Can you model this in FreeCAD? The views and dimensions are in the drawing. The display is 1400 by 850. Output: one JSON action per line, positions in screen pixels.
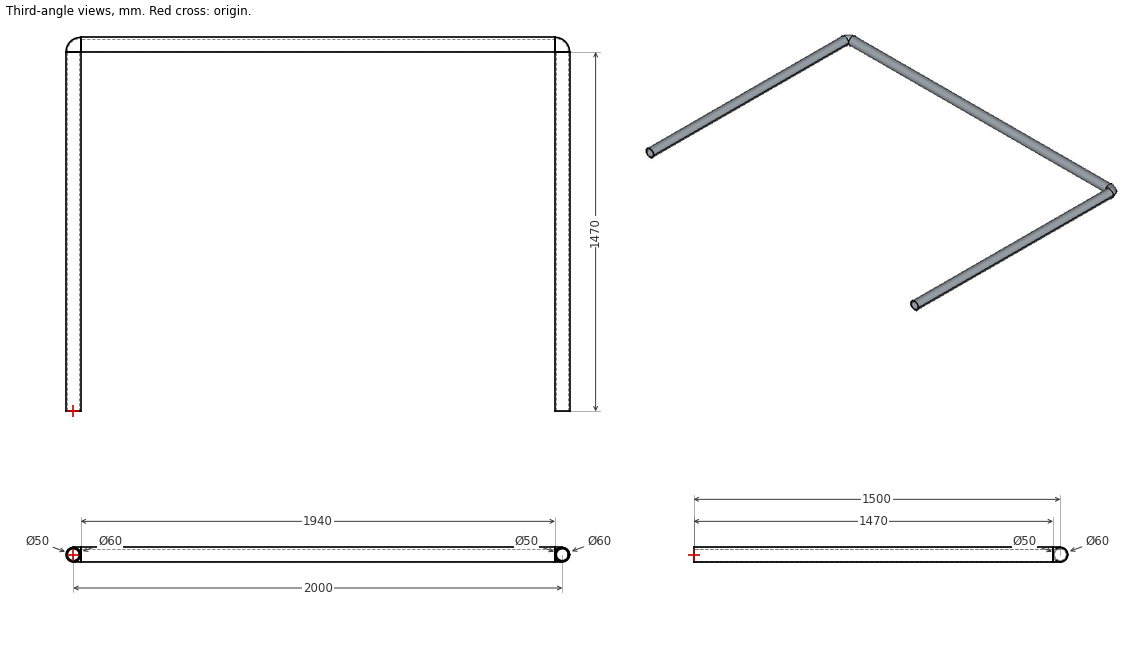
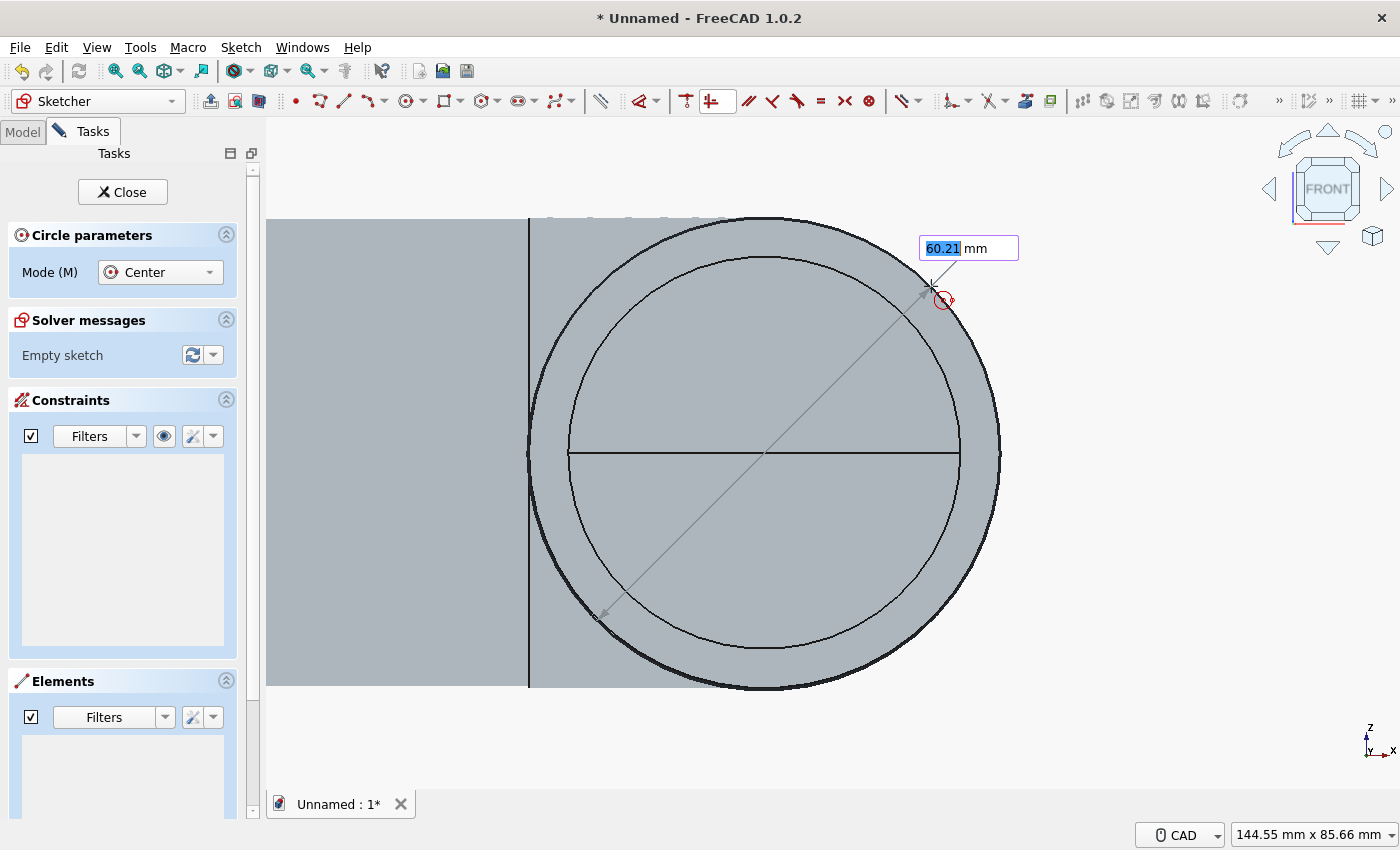
{"action": "type", "text": "60"}
{"action": "key", "text": "Return"}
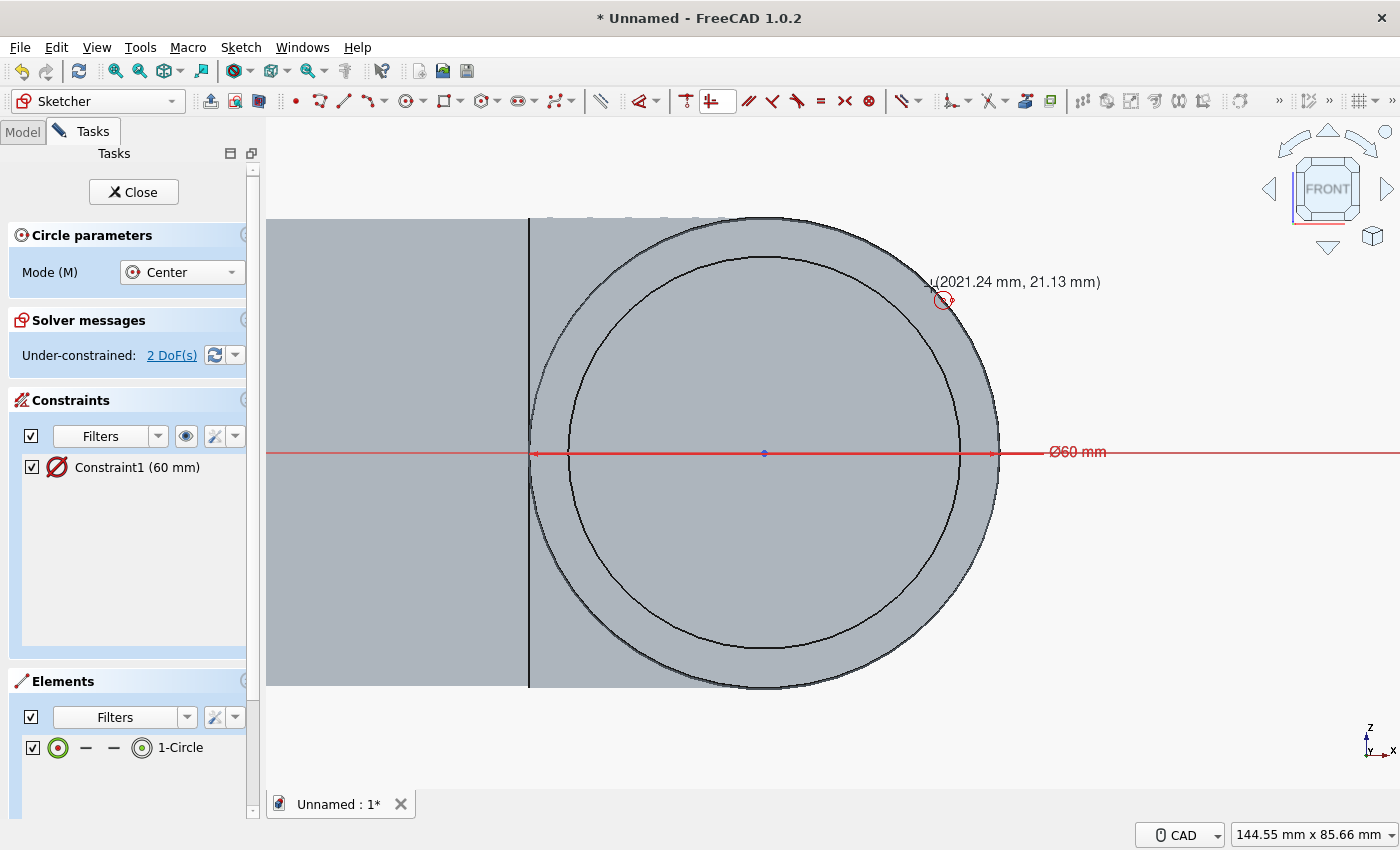
{"action": "left_click", "coordinate": [764, 454]}
{"action": "mouse_move", "coordinate": [903, 314]}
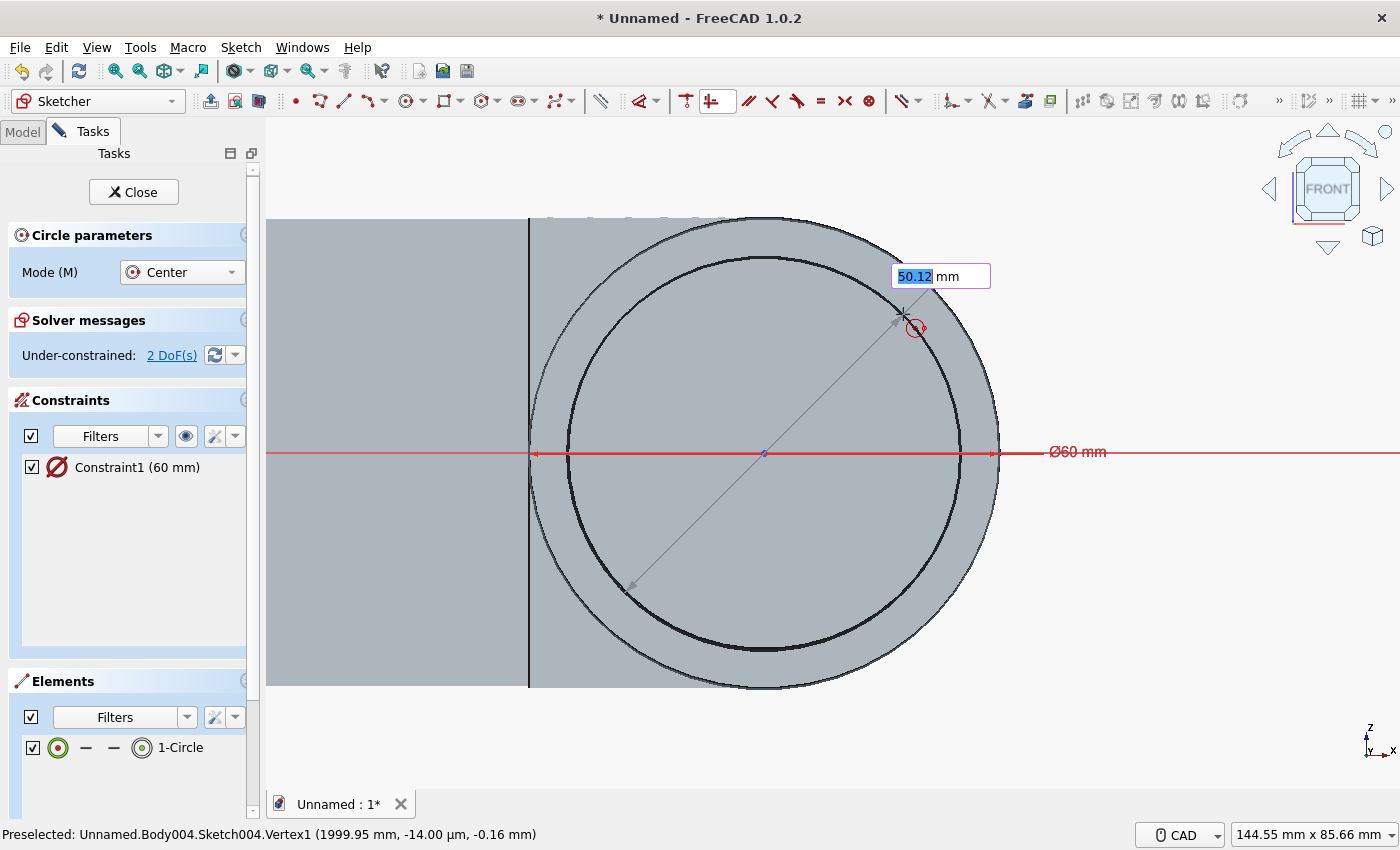
{"action": "type", "text": "50"}
{"action": "key", "text": "Return"}
{"action": "key", "text": "Escape"}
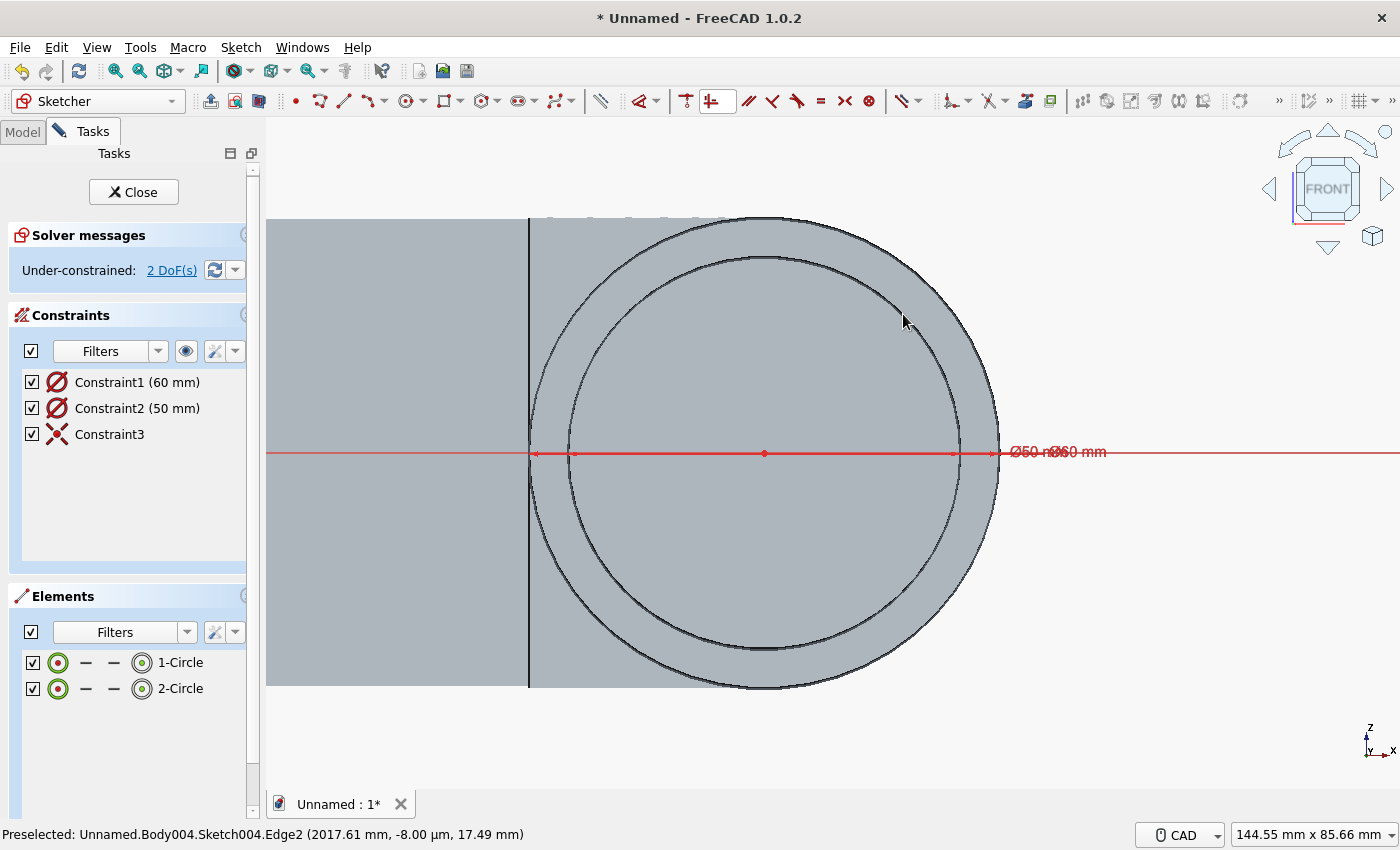
{"action": "left_click", "coordinate": [764, 454]}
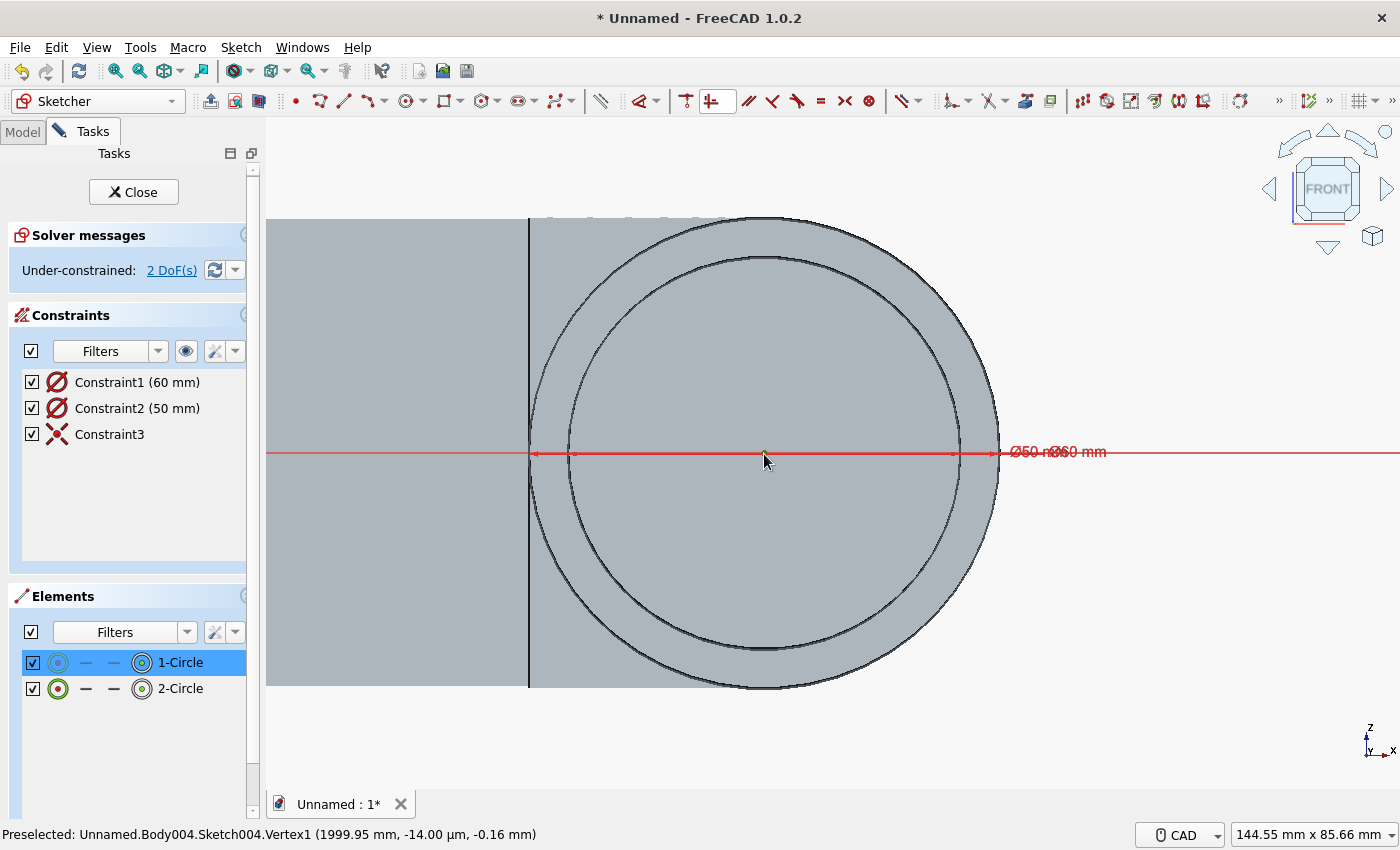
{"action": "left_click", "coordinate": [361, 453]}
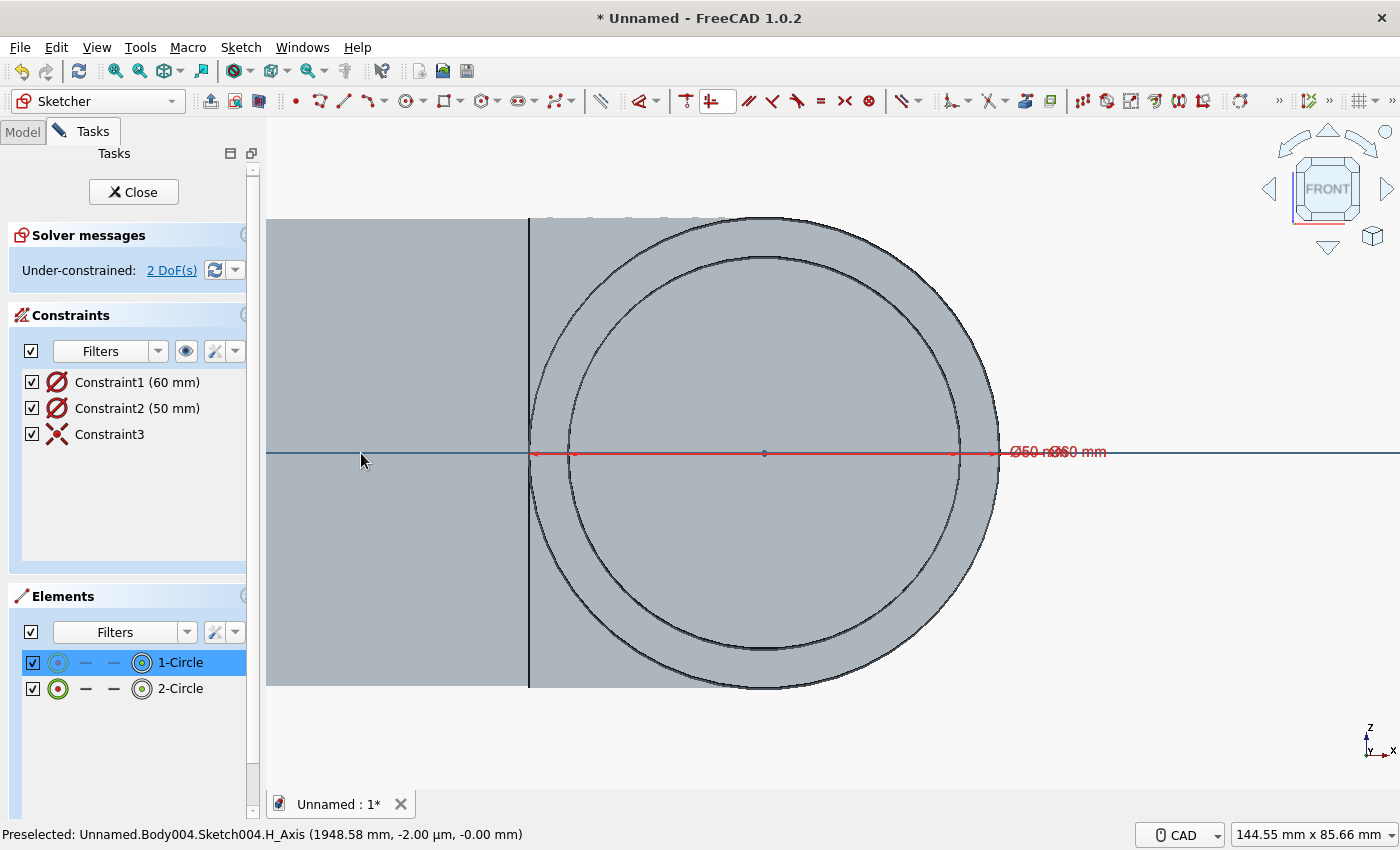
{"action": "left_click", "coordinate": [686, 102]}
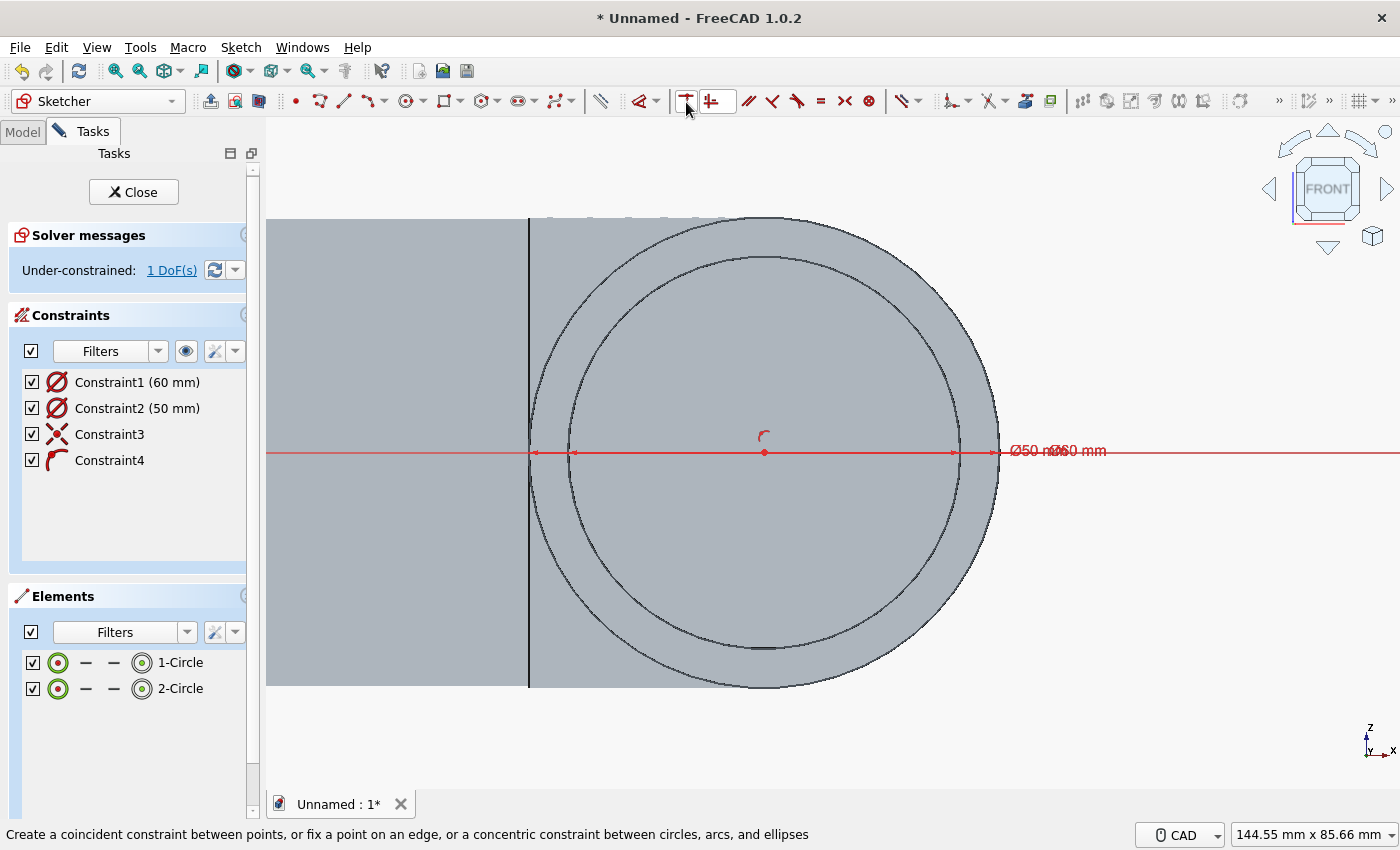
{"action": "left_click", "coordinate": [640, 102]}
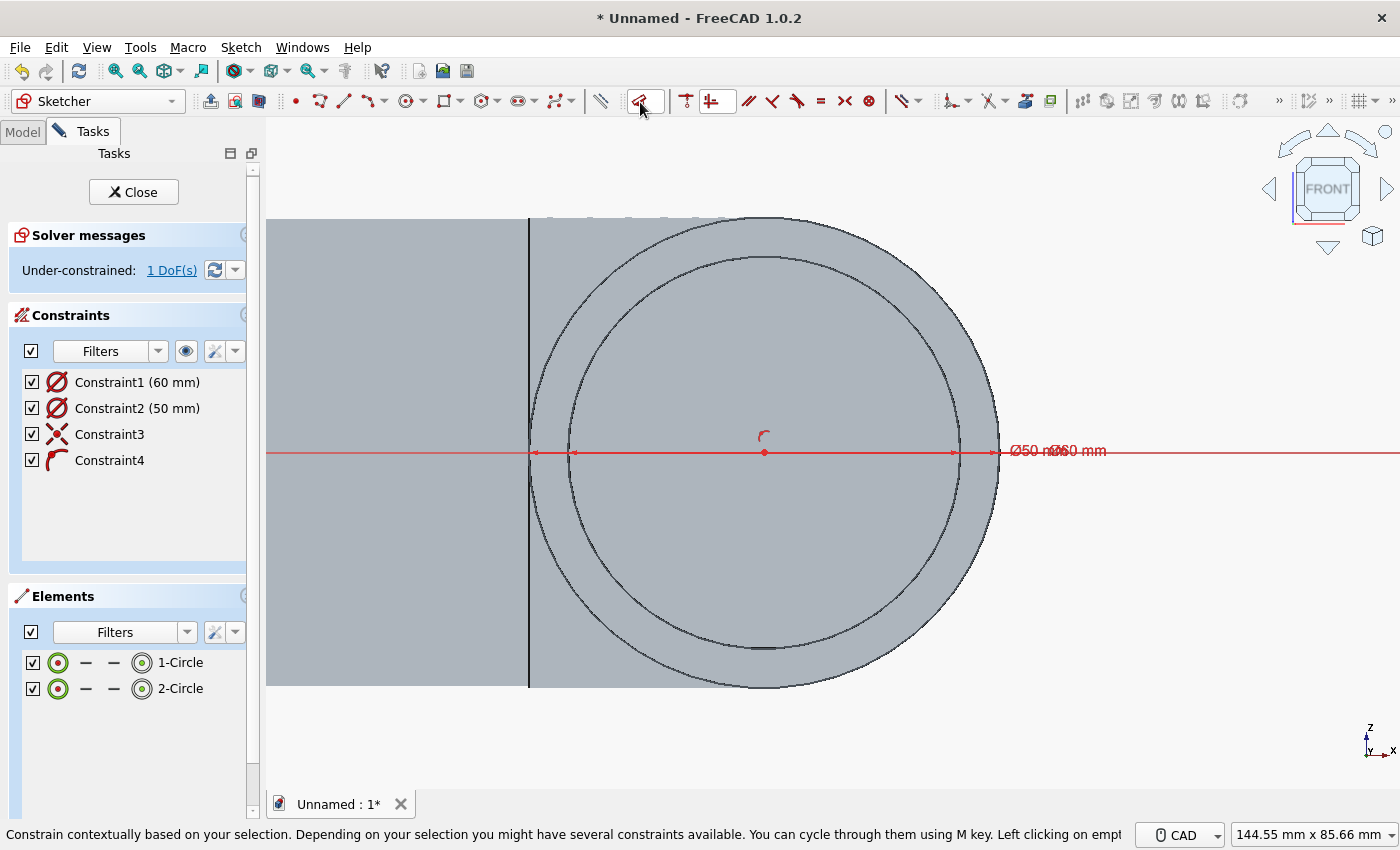
{"action": "left_click", "coordinate": [764, 453]}
{"action": "left_click", "coordinate": [421, 487]}